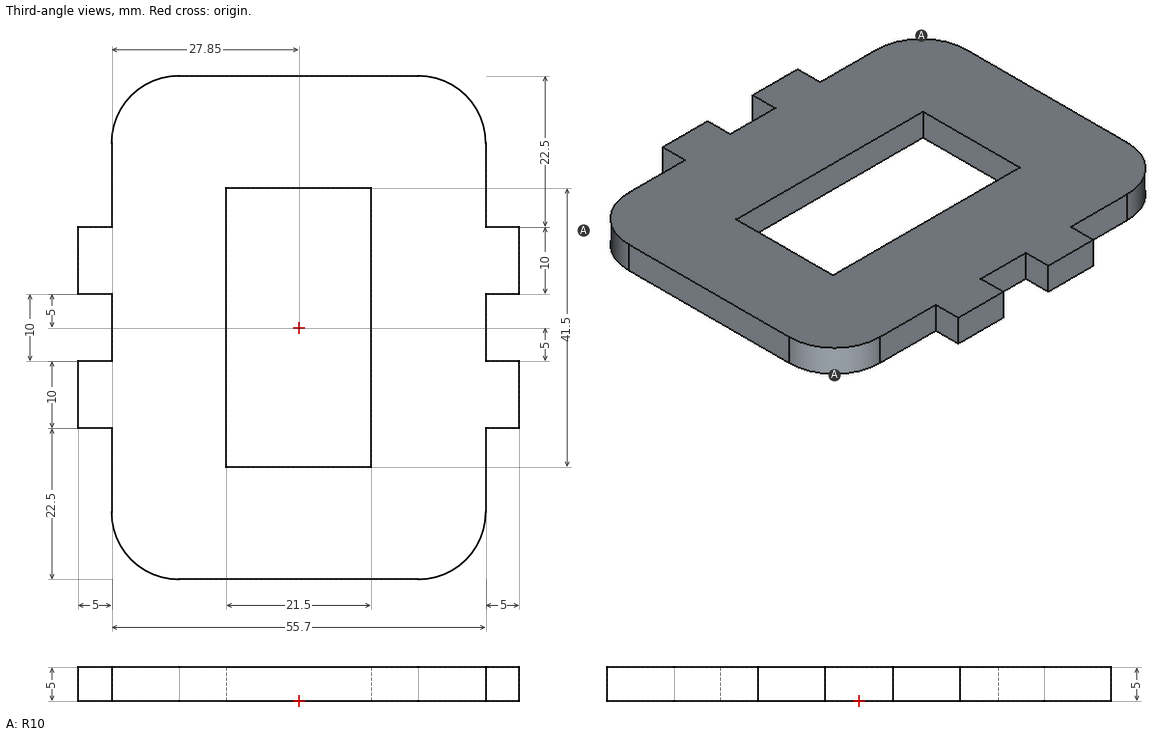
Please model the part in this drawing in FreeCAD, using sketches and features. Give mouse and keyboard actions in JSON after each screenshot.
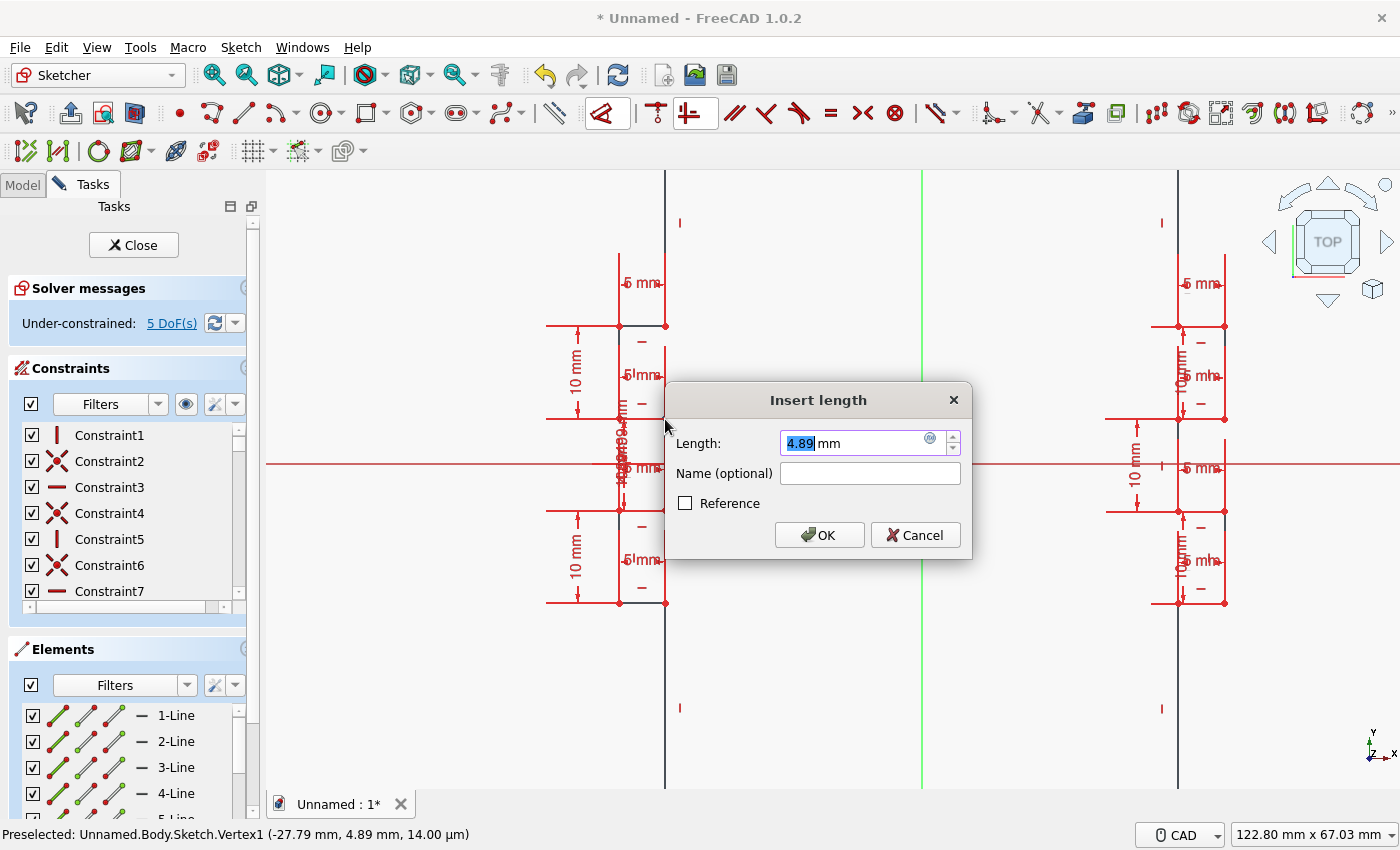
{"action": "type", "text": "5"}
{"action": "key", "text": "Return"}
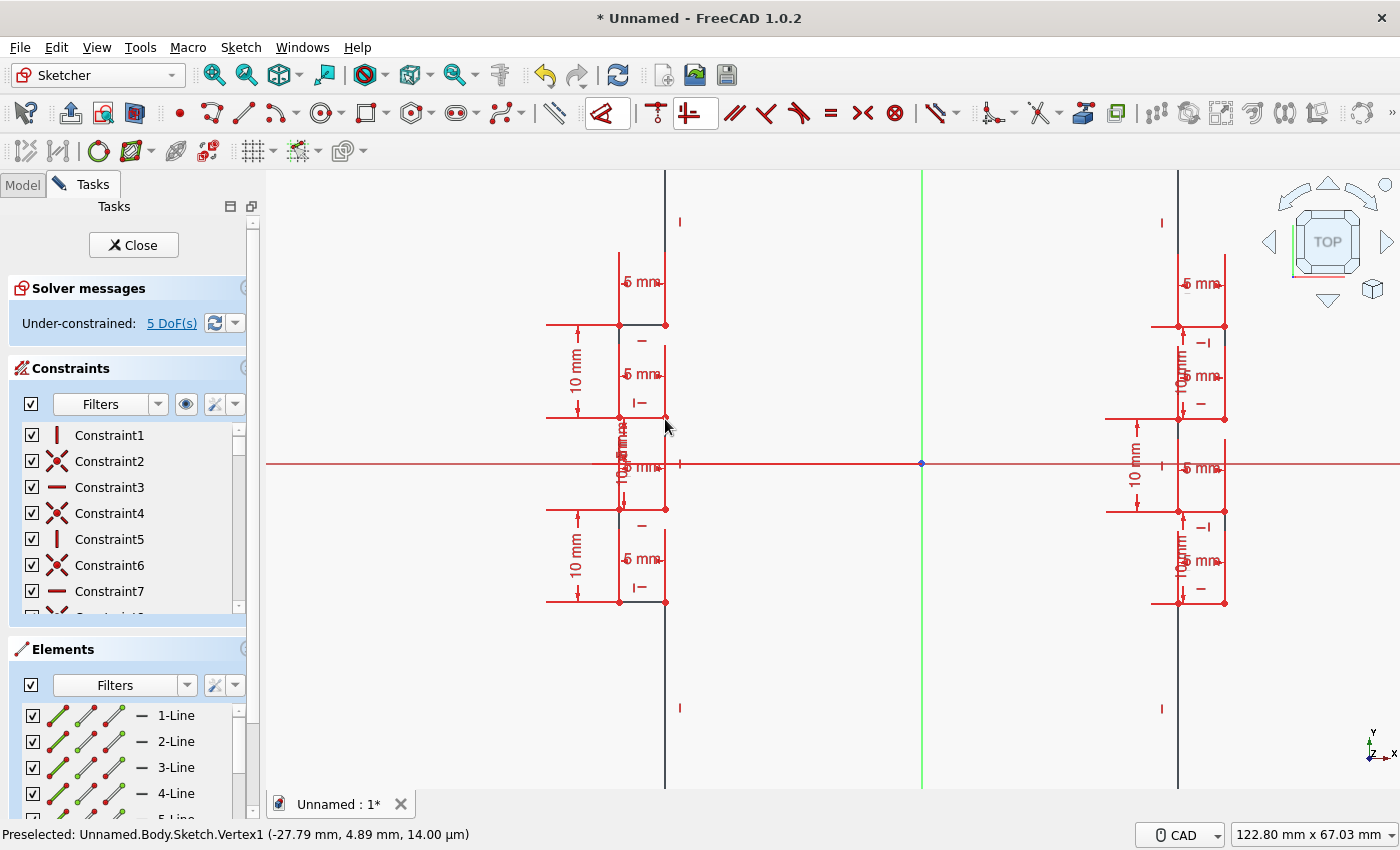
{"action": "left_click", "coordinate": [1225, 512]}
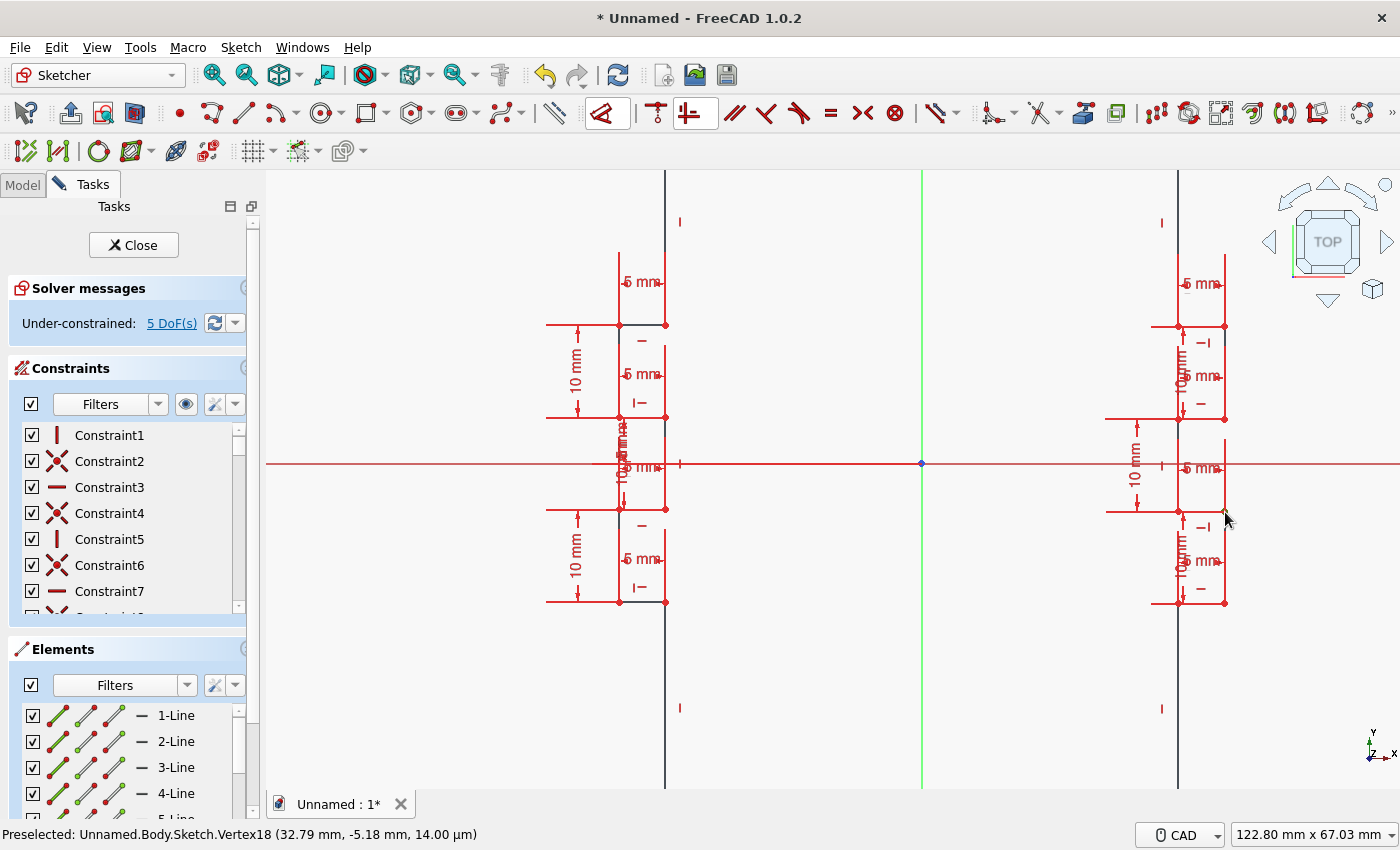
{"action": "key", "text": "i"}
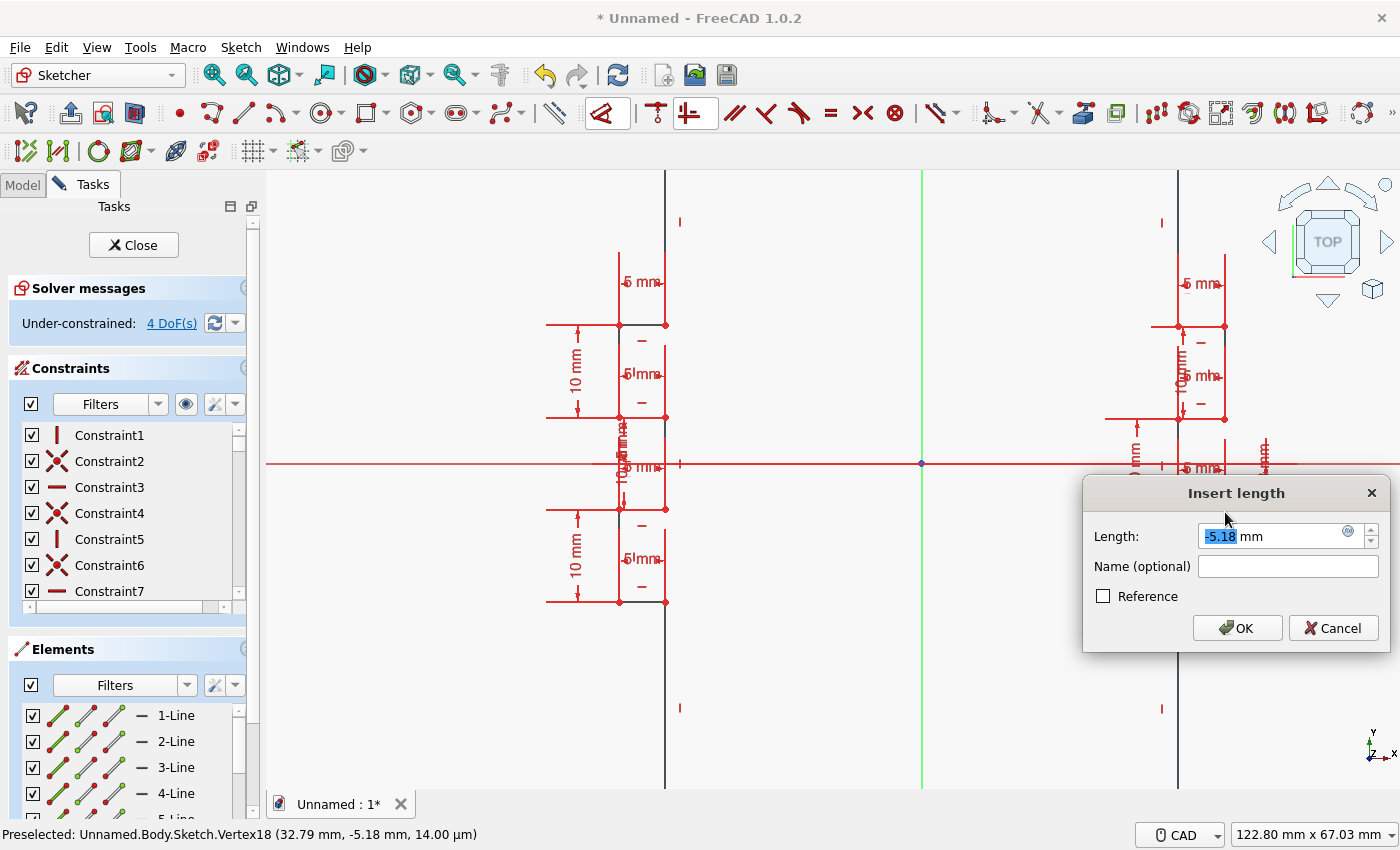
{"action": "type", "text": "-5"}
{"action": "key", "text": "Return"}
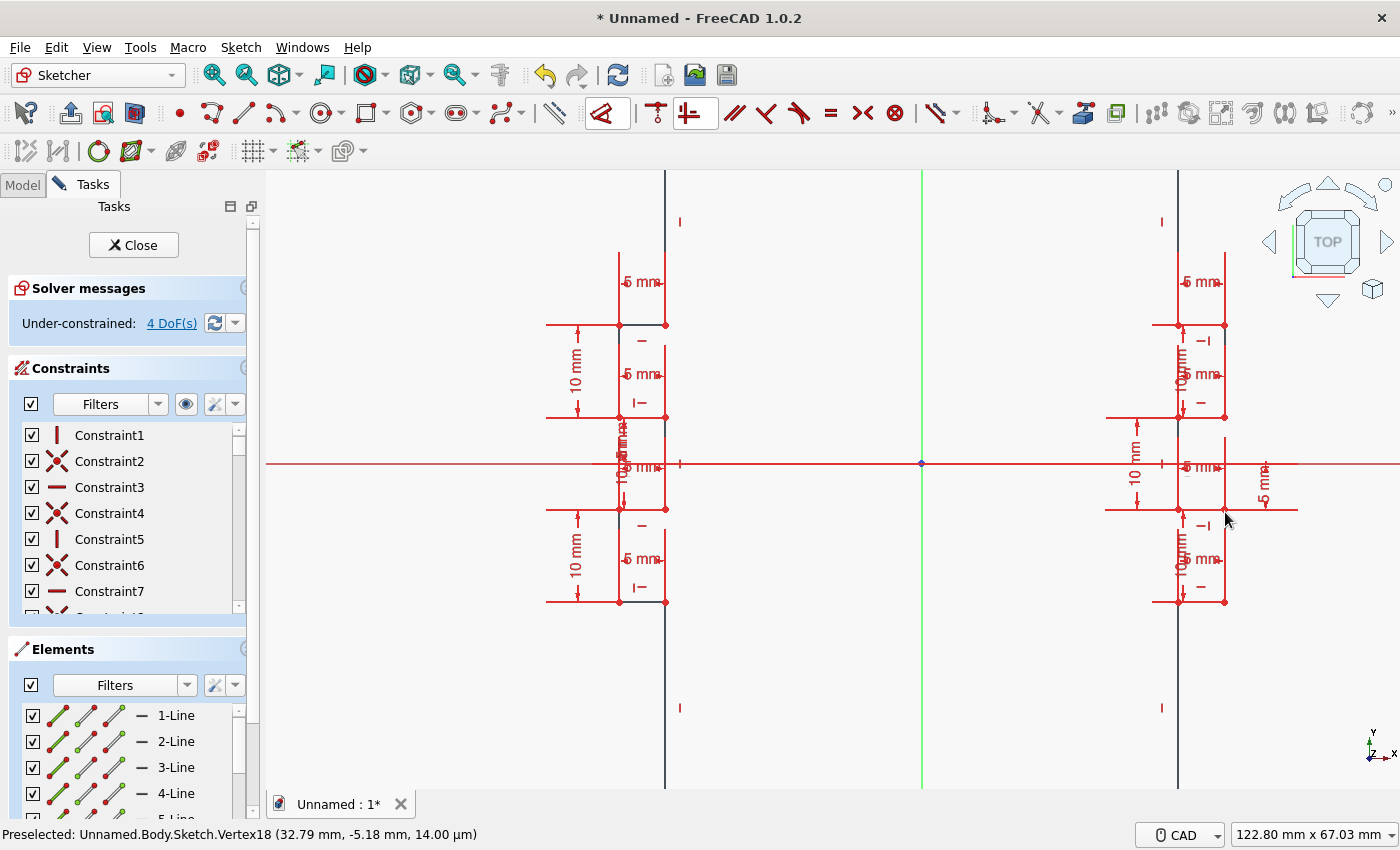
{"action": "left_click", "coordinate": [665, 665]}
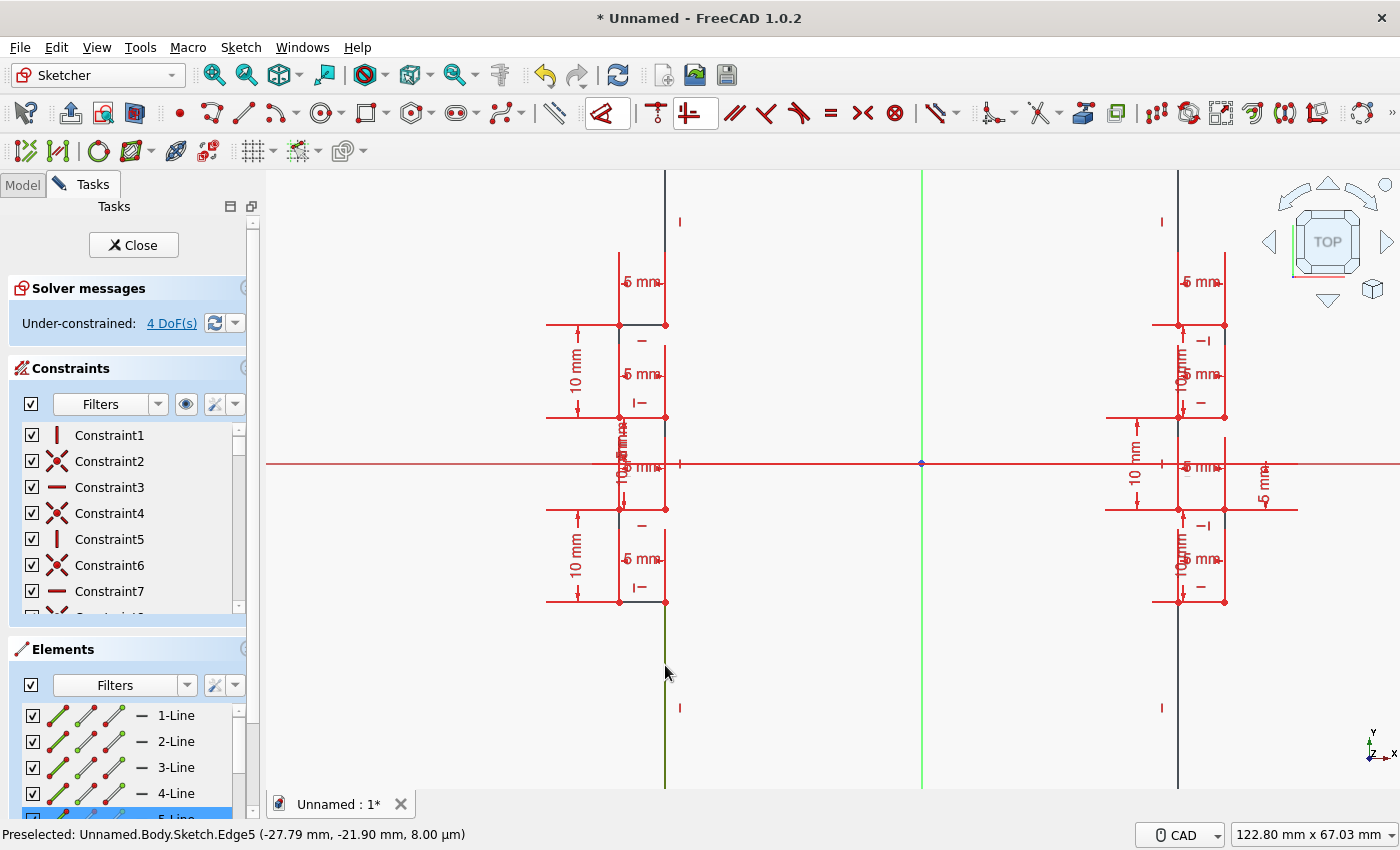
{"action": "key", "text": "i"}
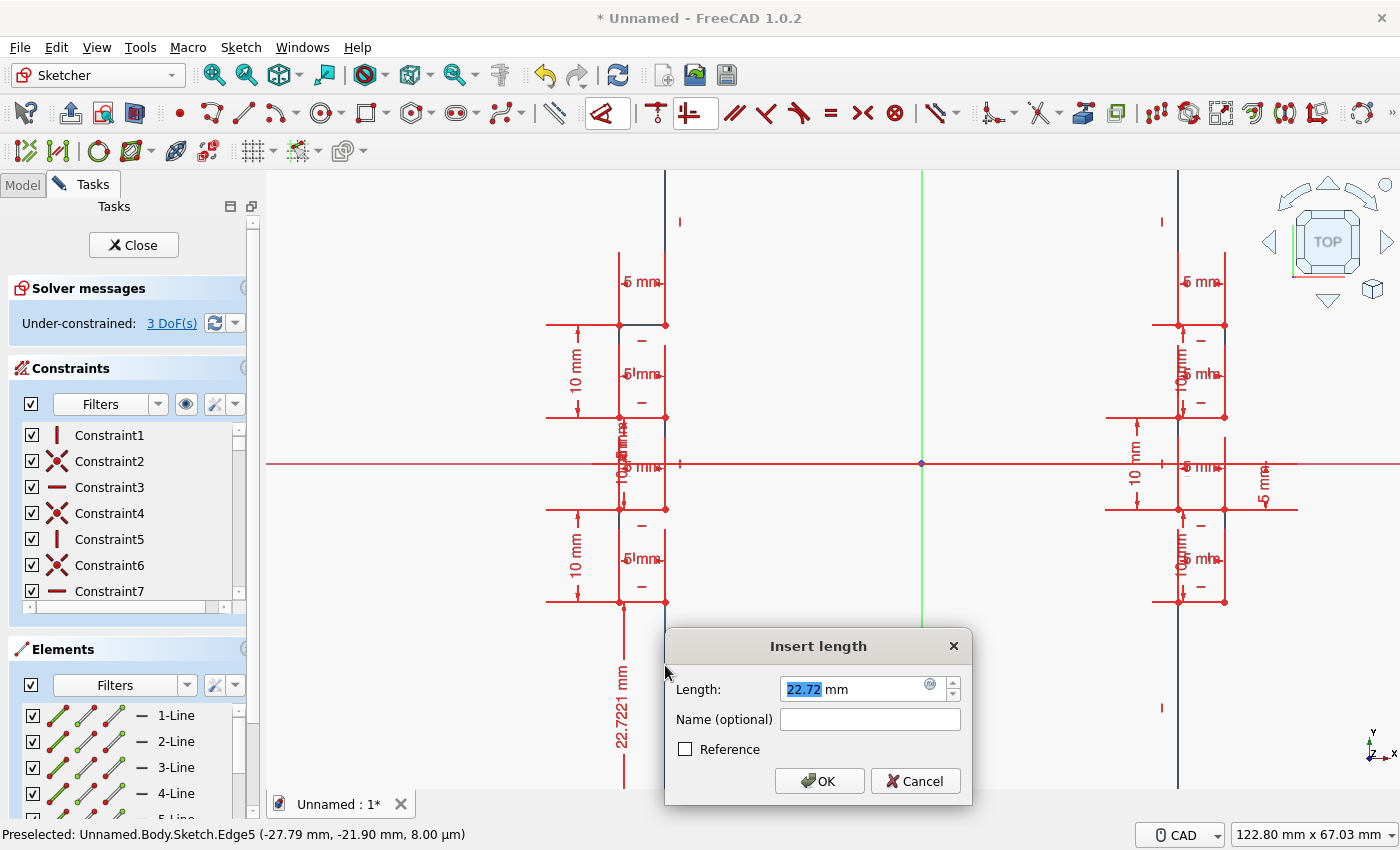
{"action": "type", "text": "22.5"}
{"action": "key", "text": "Return"}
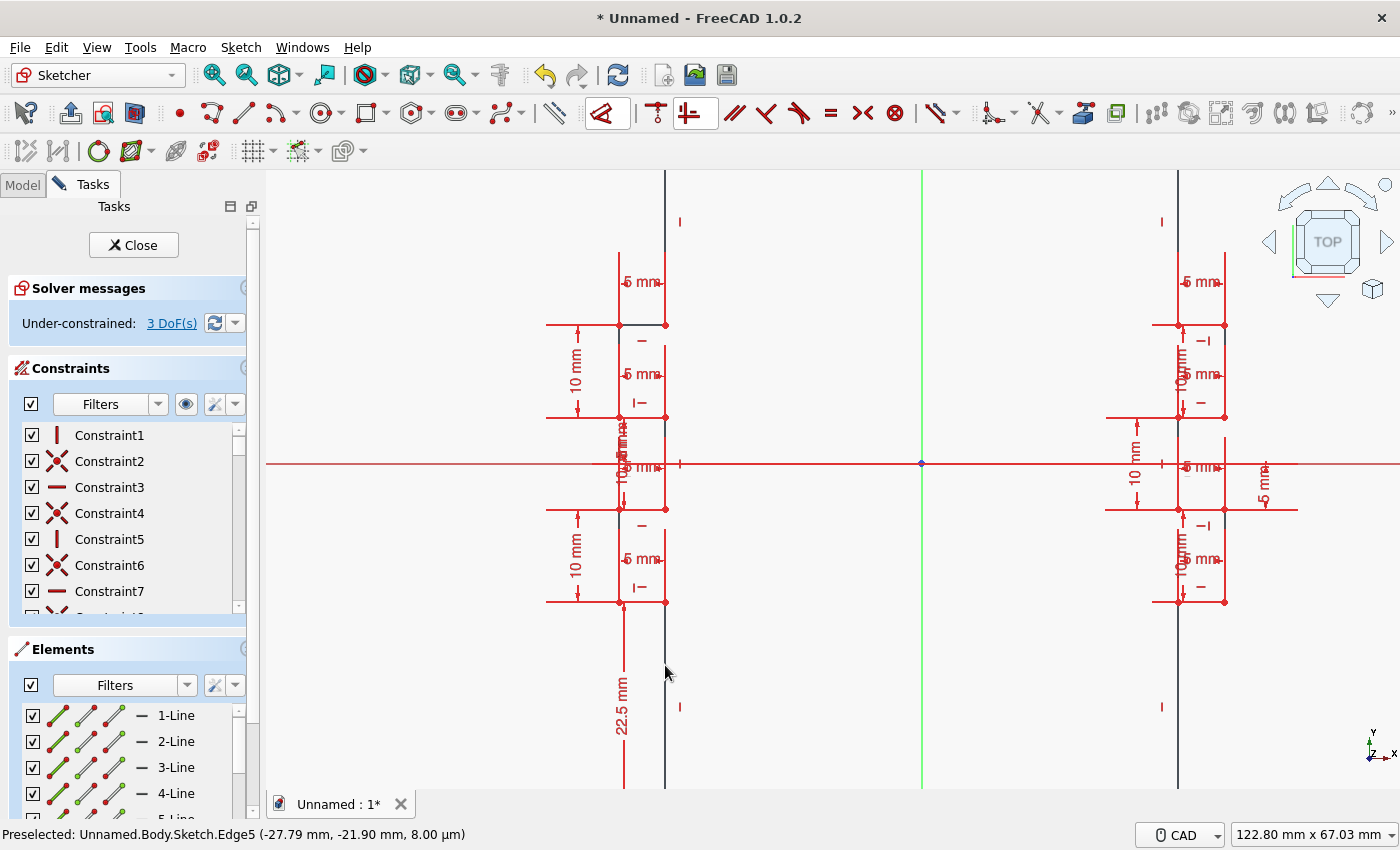
{"action": "scroll", "coordinate": [573, 499], "scroll_direction": "down", "scroll_amount": 3}